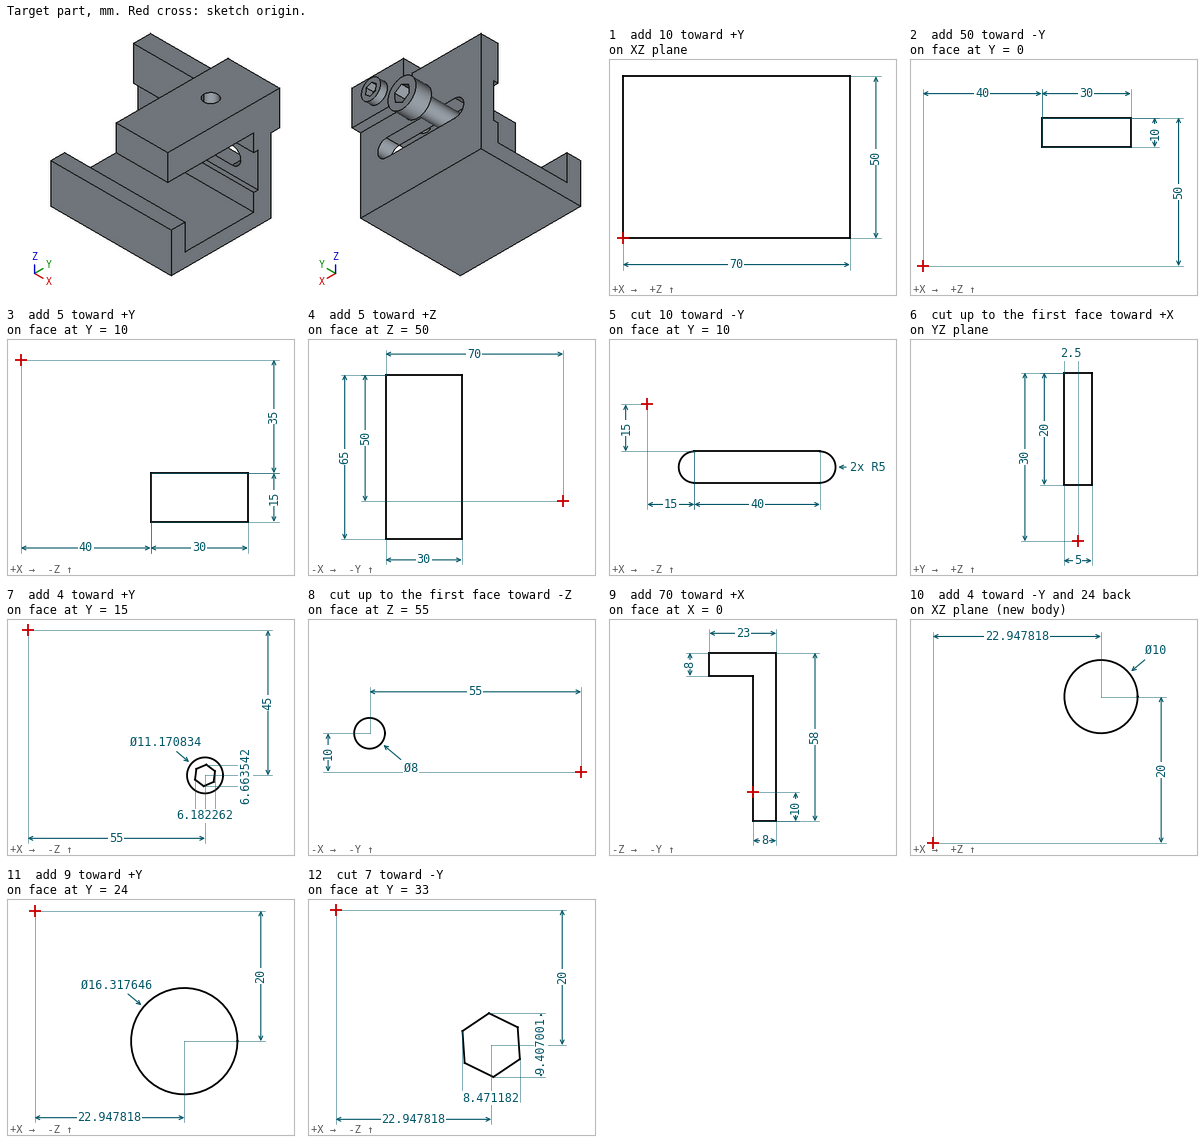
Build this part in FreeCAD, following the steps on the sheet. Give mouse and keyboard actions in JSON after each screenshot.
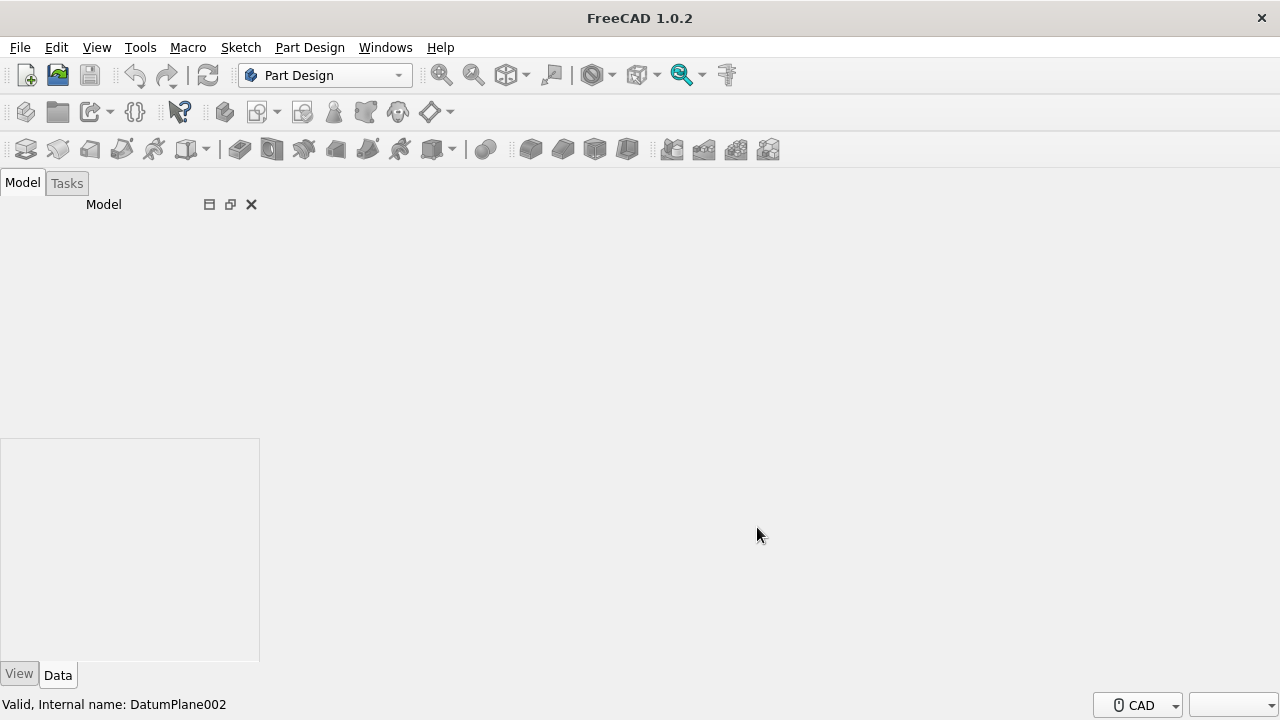
{"action": "left_click", "coordinate": [26, 76]}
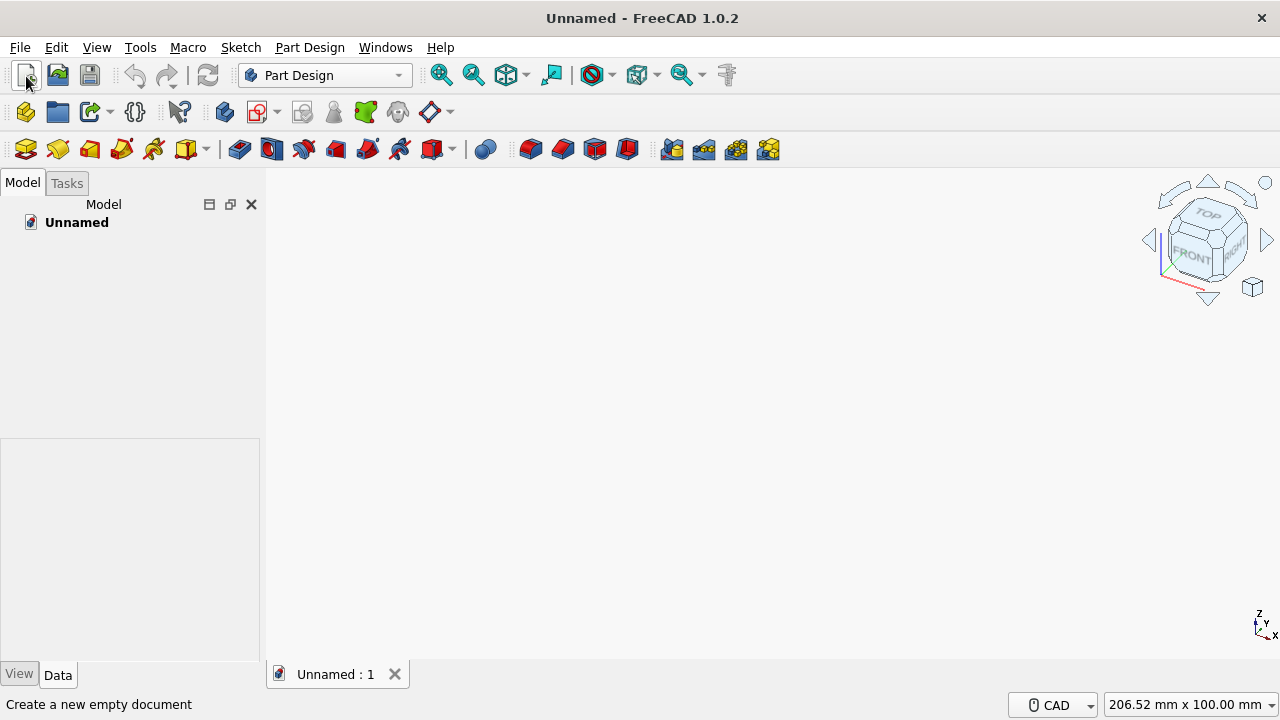
{"action": "left_click", "coordinate": [258, 112]}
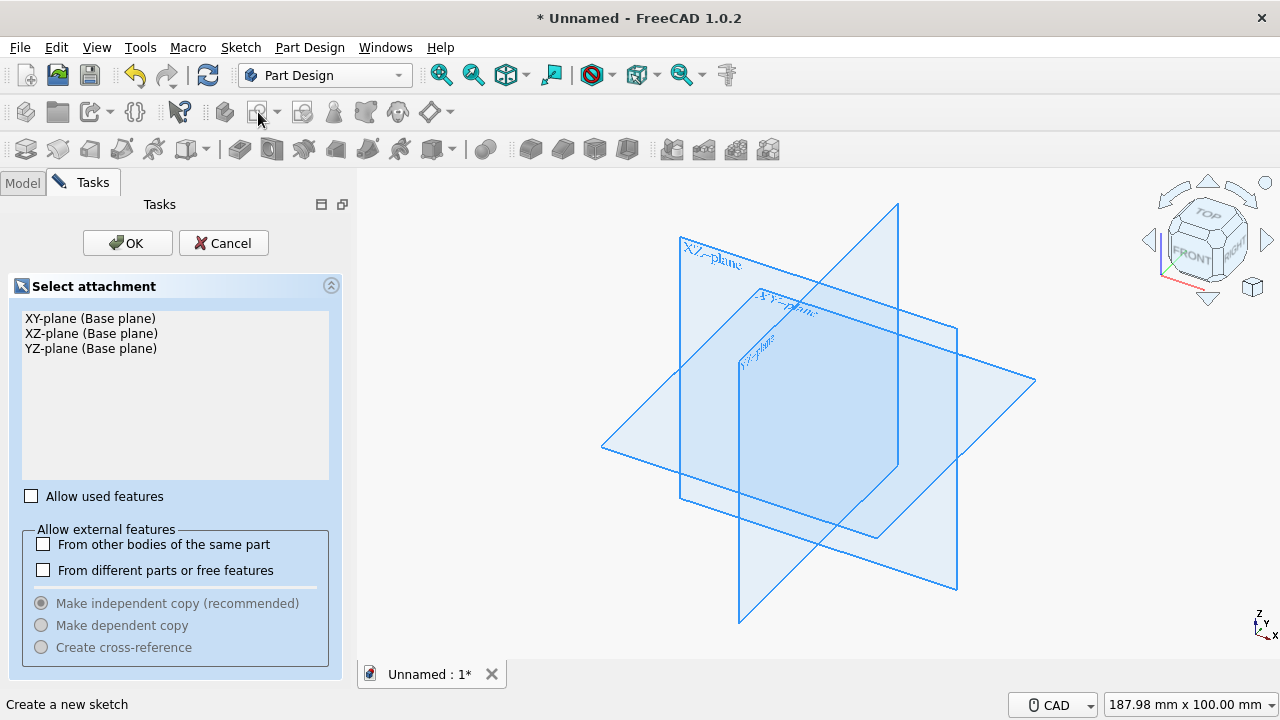
{"action": "left_click", "coordinate": [82, 334]}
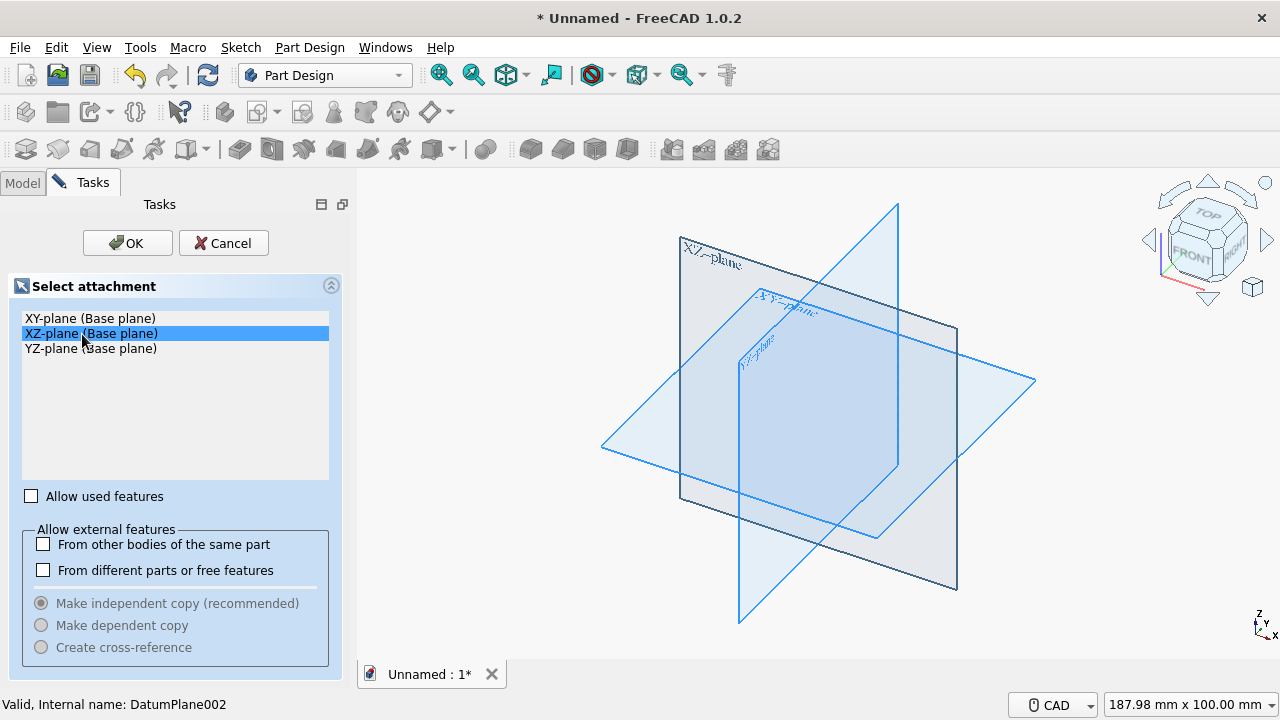
{"action": "left_click", "coordinate": [128, 243]}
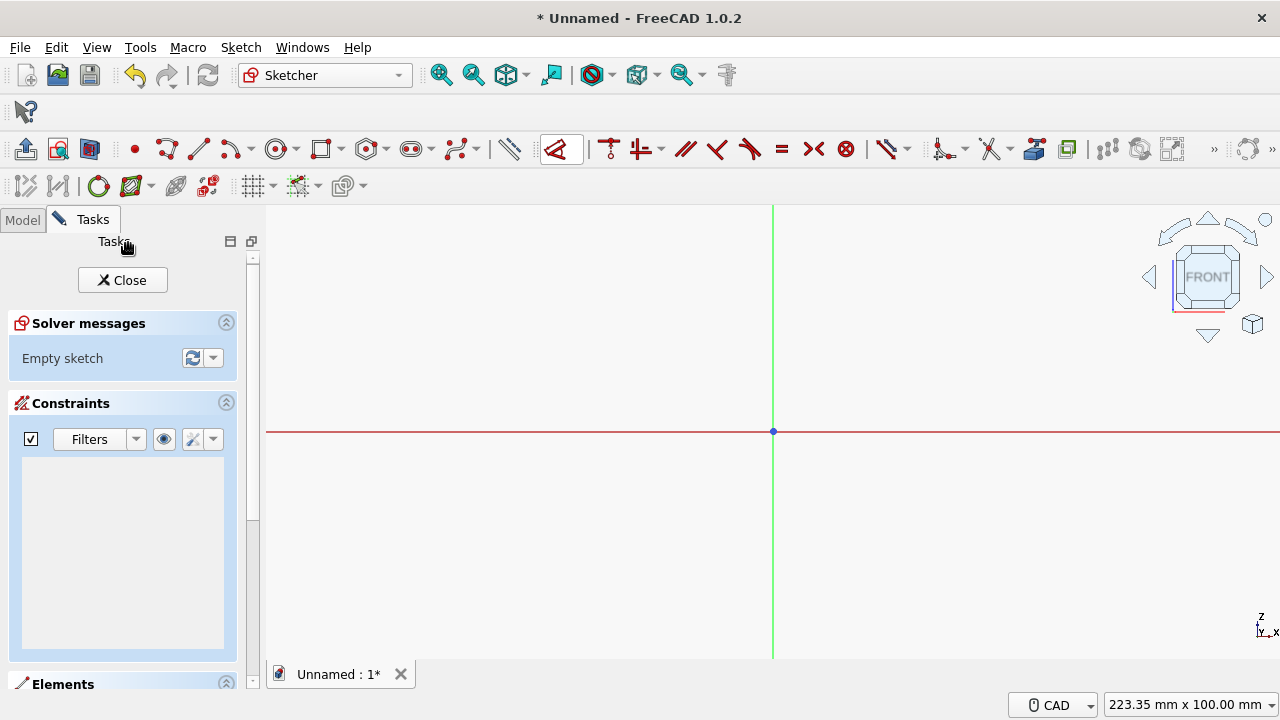
{"action": "scroll", "coordinate": [294, 631], "scroll_direction": "down", "scroll_amount": 1}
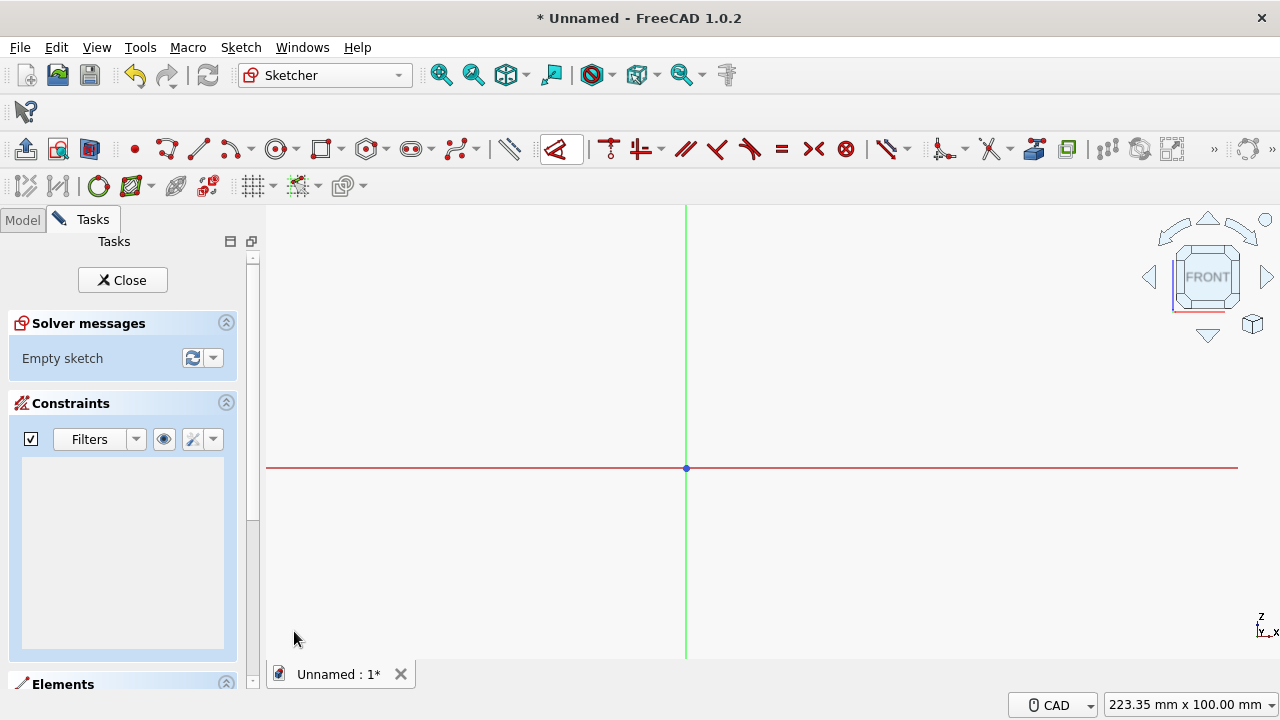
{"action": "scroll", "coordinate": [1044, 260], "scroll_direction": "up", "scroll_amount": 2}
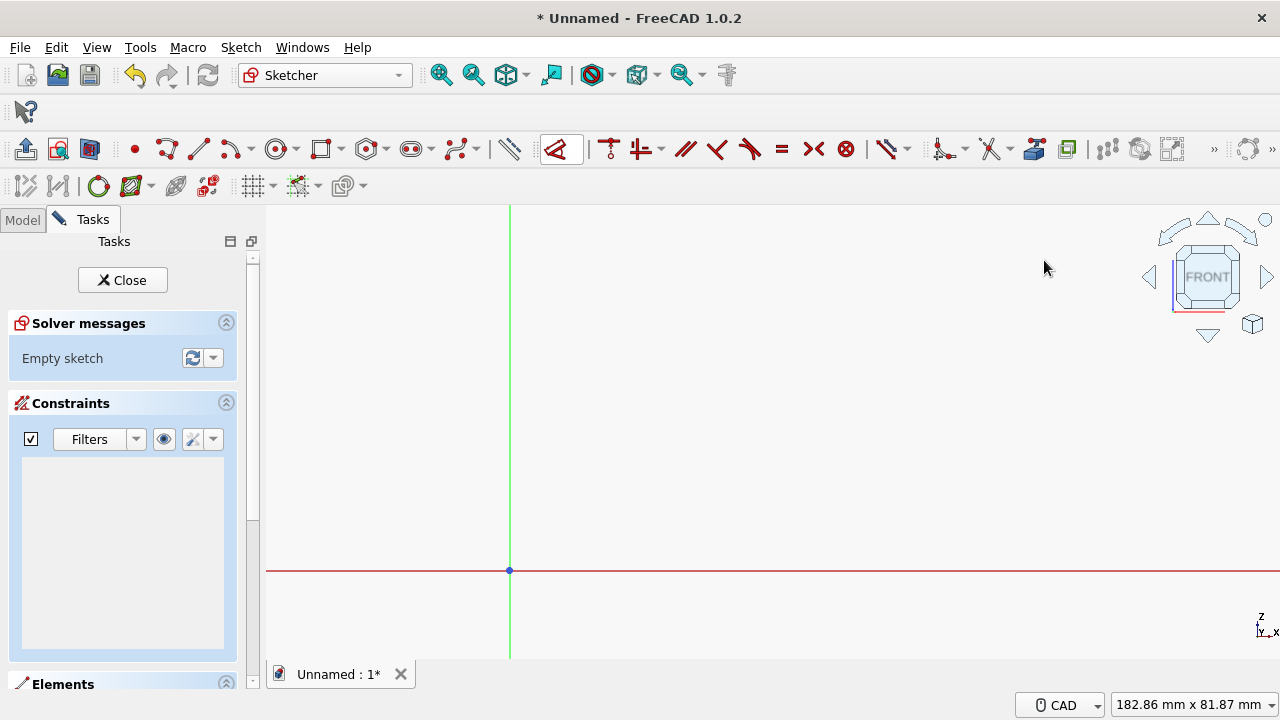
{"action": "left_click", "coordinate": [322, 150]}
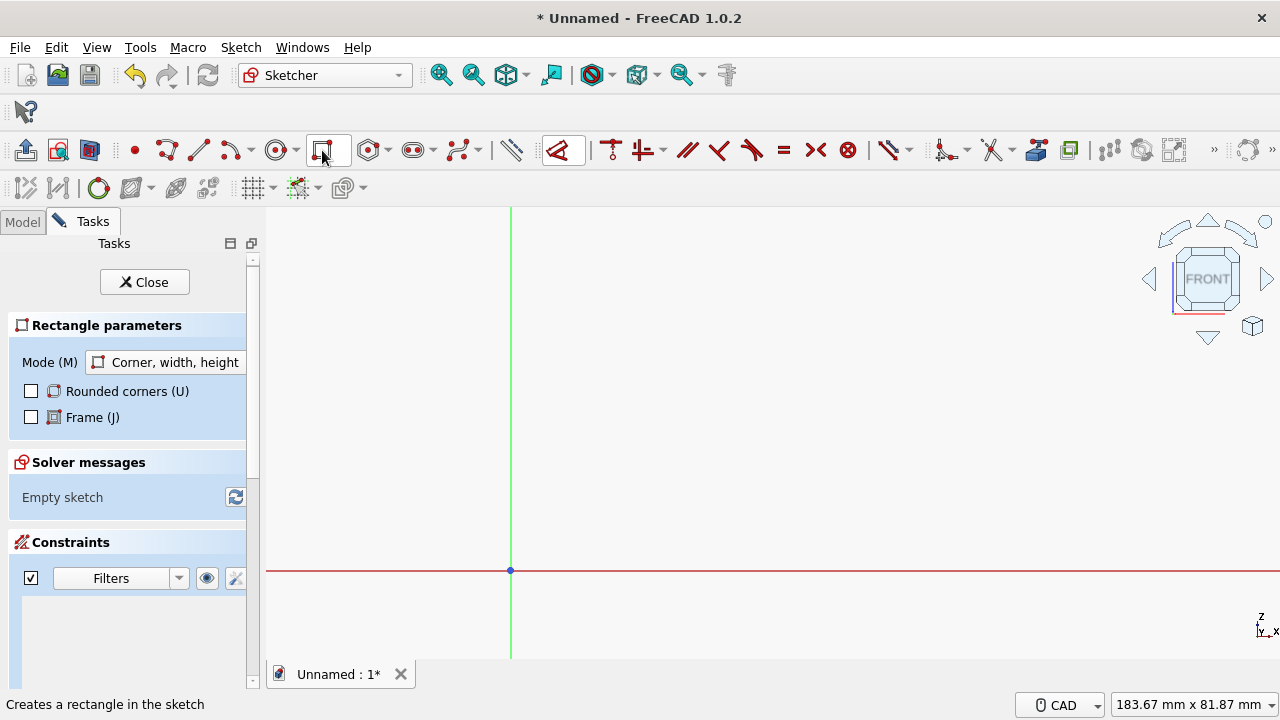
{"action": "left_click", "coordinate": [511, 571]}
{"action": "left_click", "coordinate": [897, 295]}
{"action": "key", "text": "Escape"}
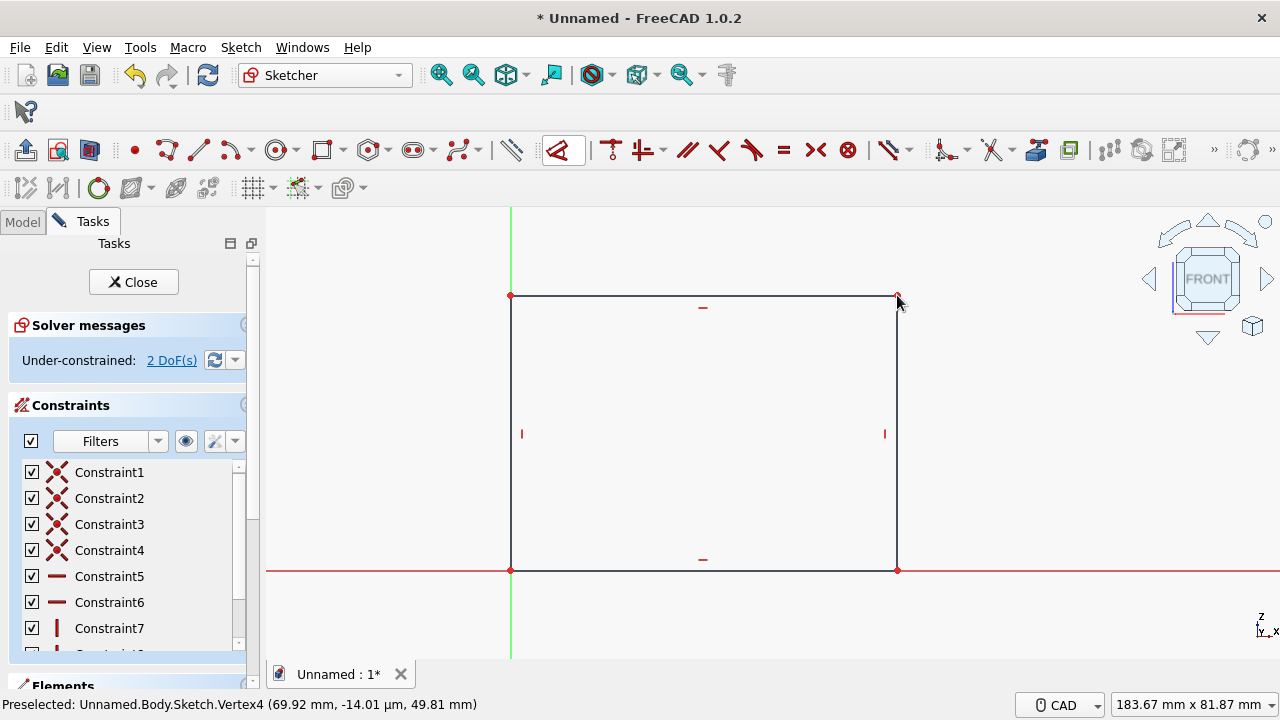
{"action": "left_click", "coordinate": [558, 150]}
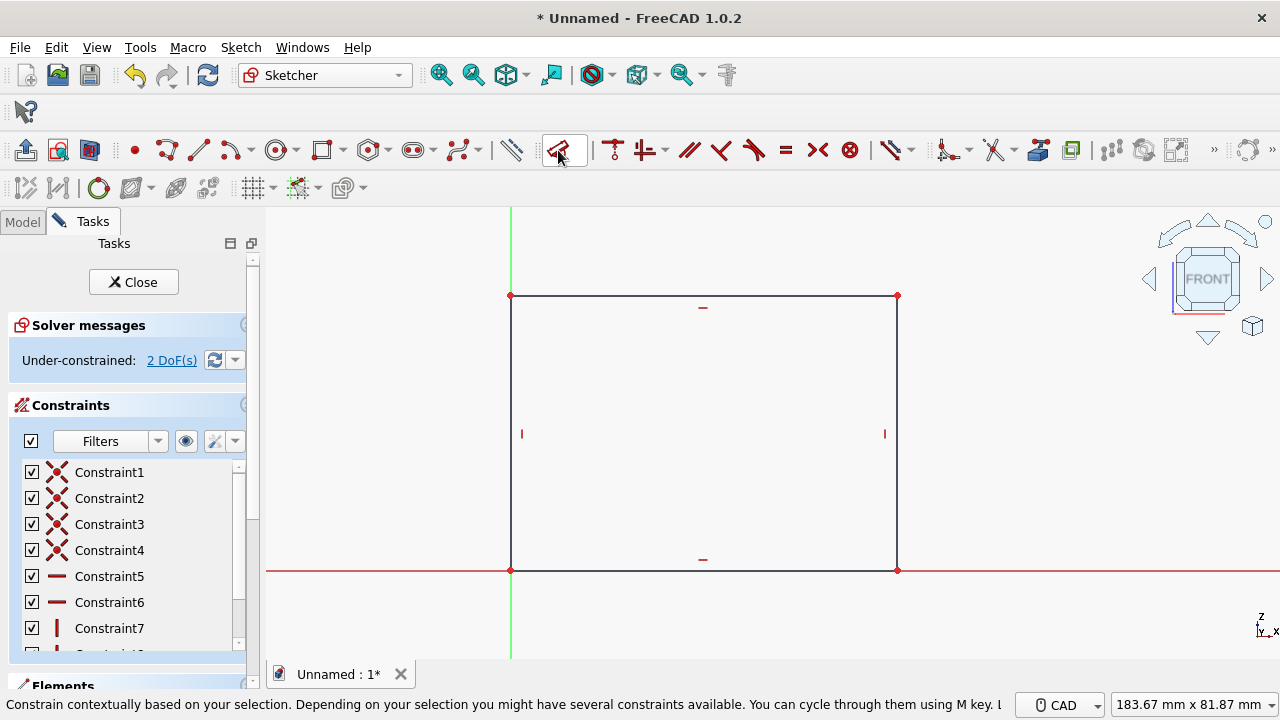
{"action": "left_click", "coordinate": [627, 571]}
{"action": "left_click", "coordinate": [704, 605]}